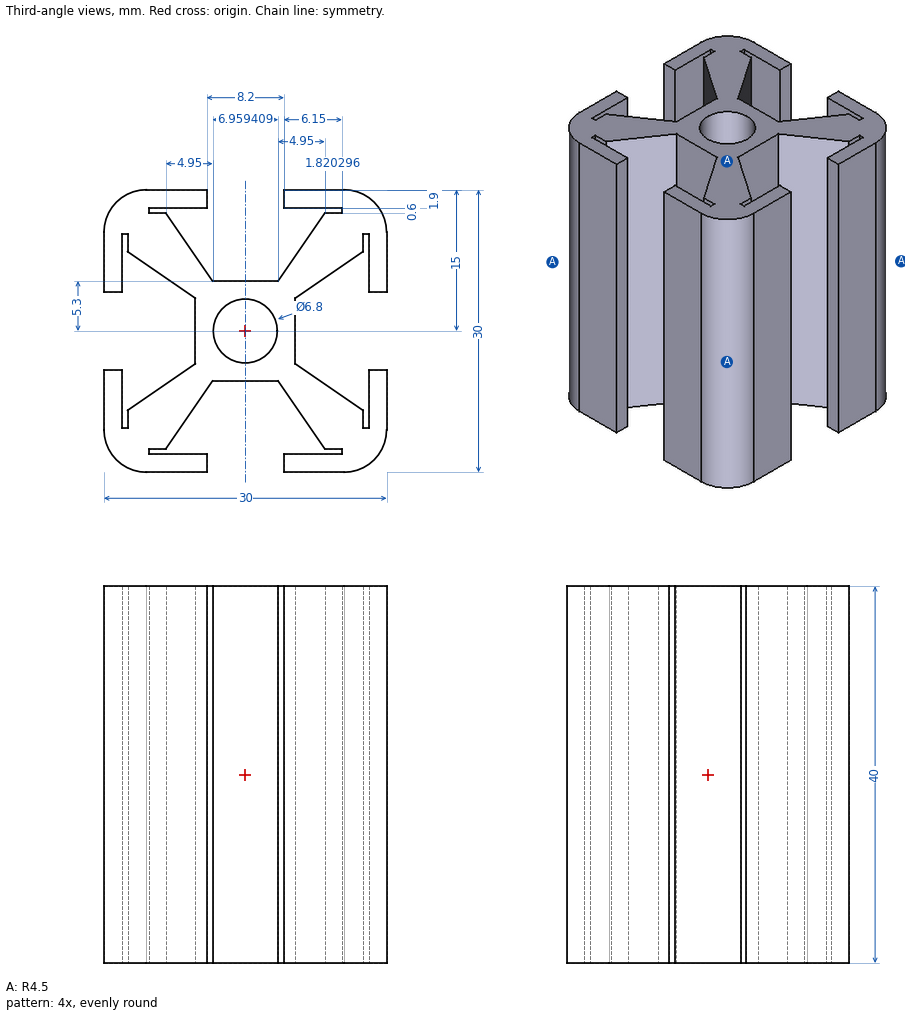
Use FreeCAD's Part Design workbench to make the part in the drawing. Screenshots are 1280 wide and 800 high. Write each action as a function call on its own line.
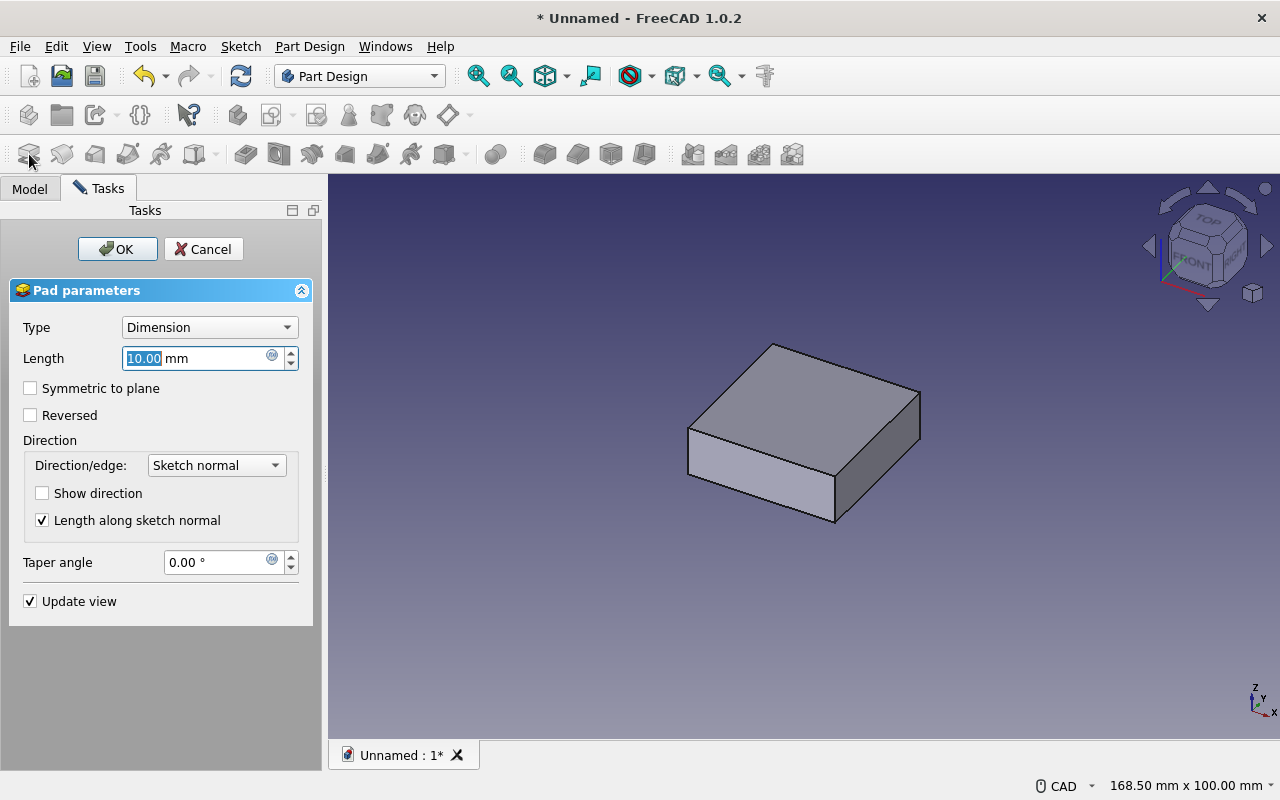
text(40)
key(Tab)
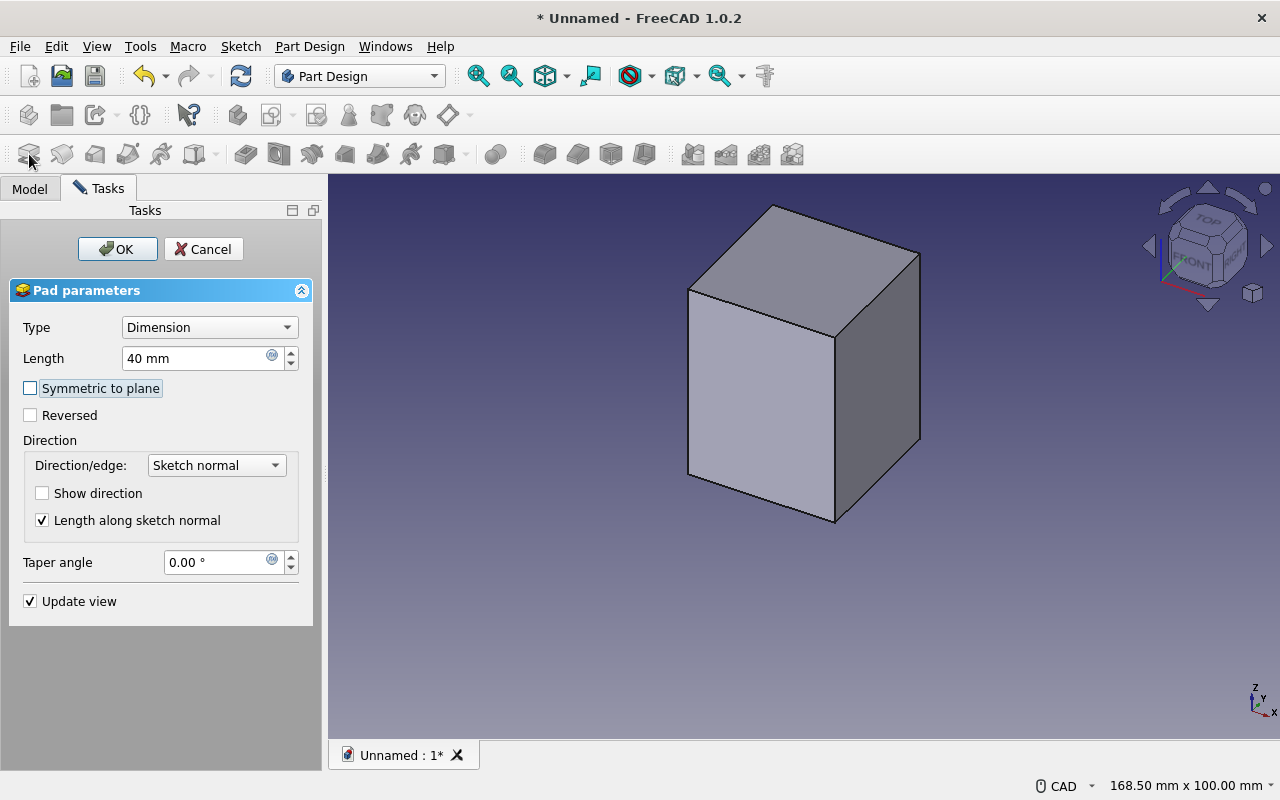
click(31, 388)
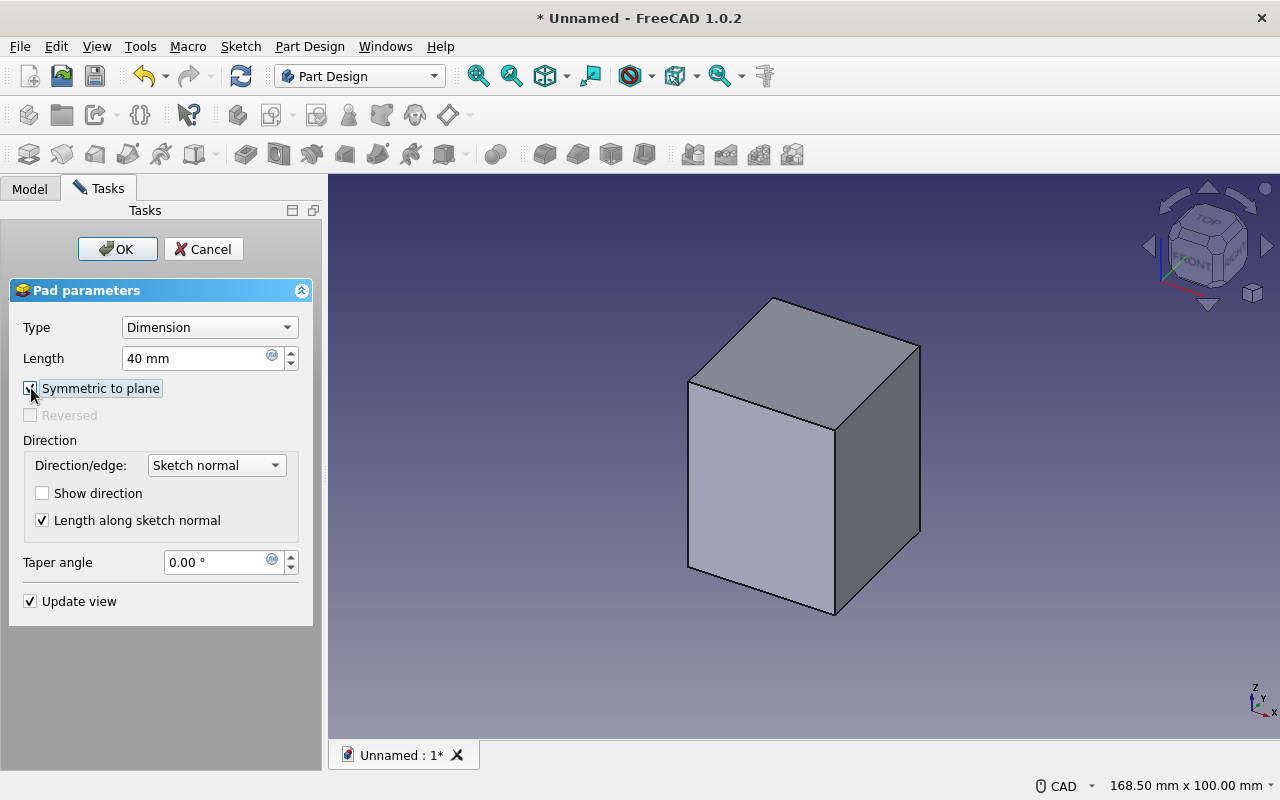
click(118, 249)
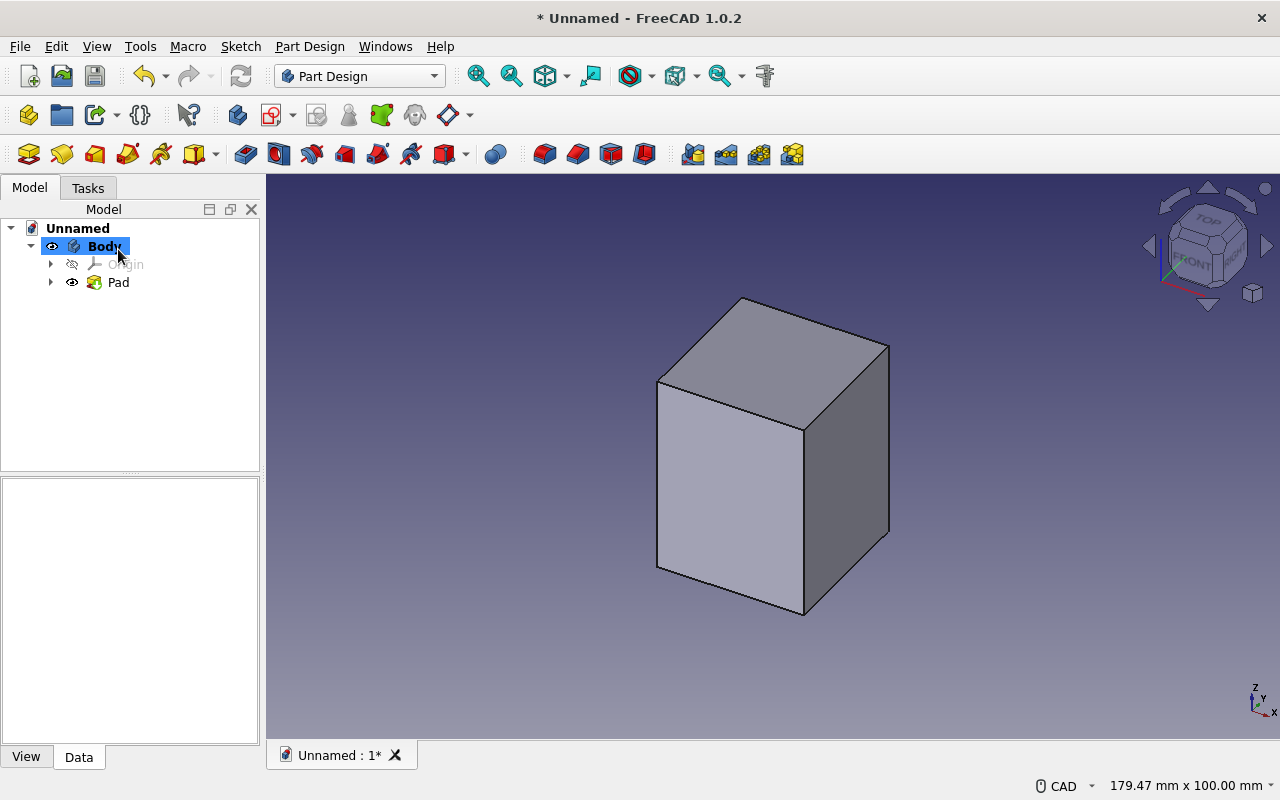
click(804, 522)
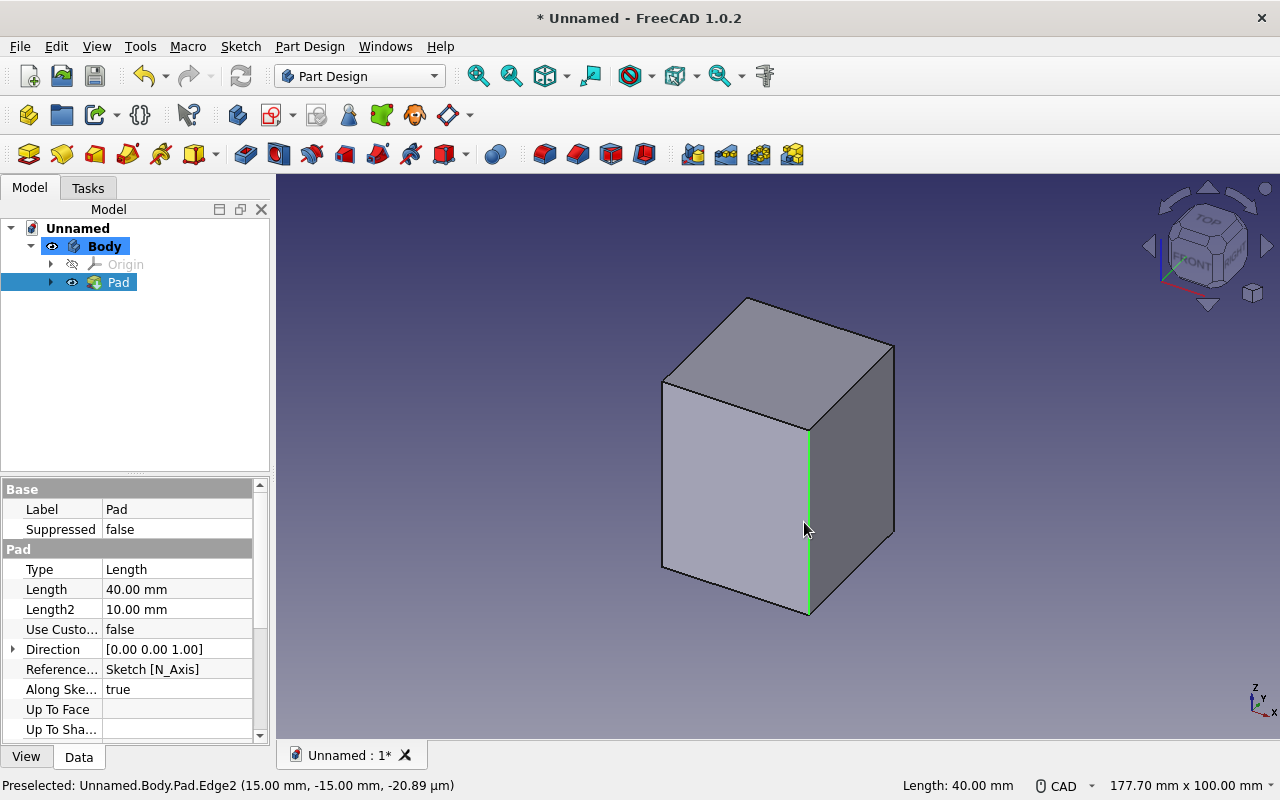
key(0)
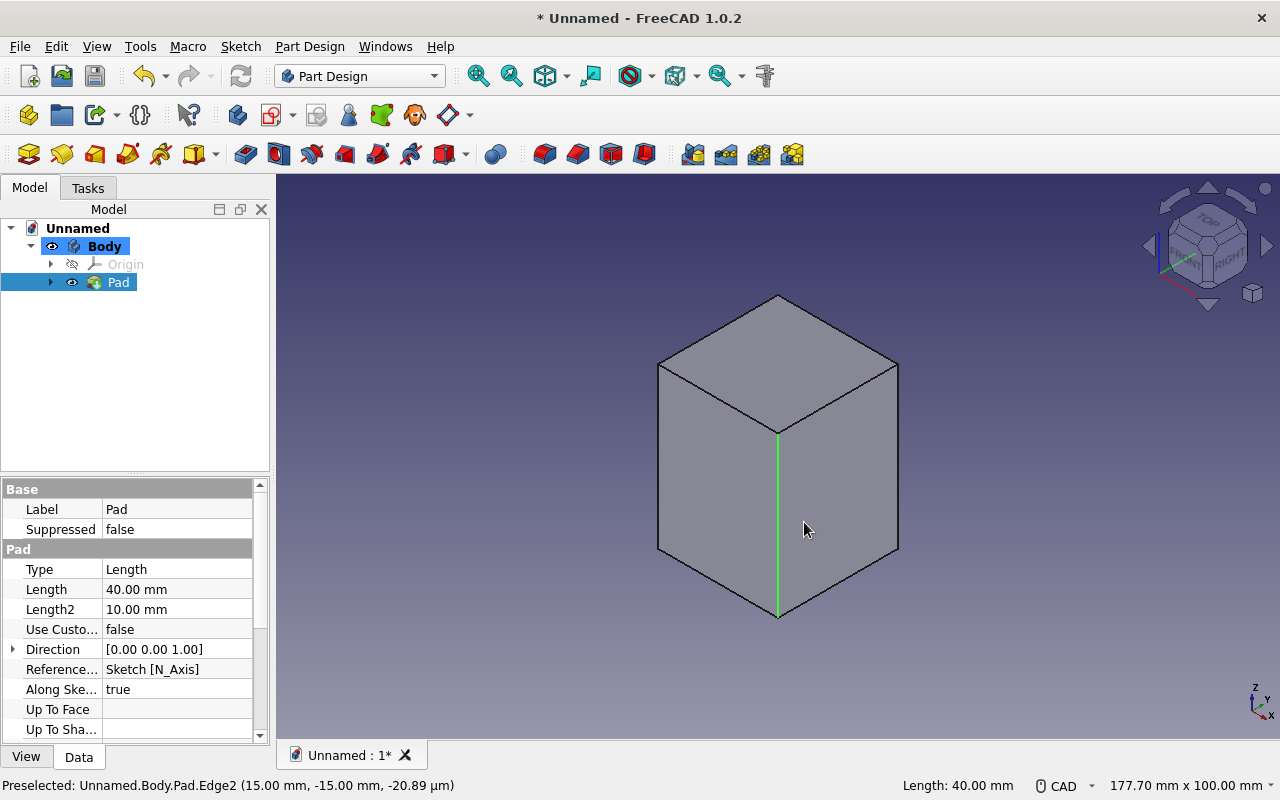
key(2)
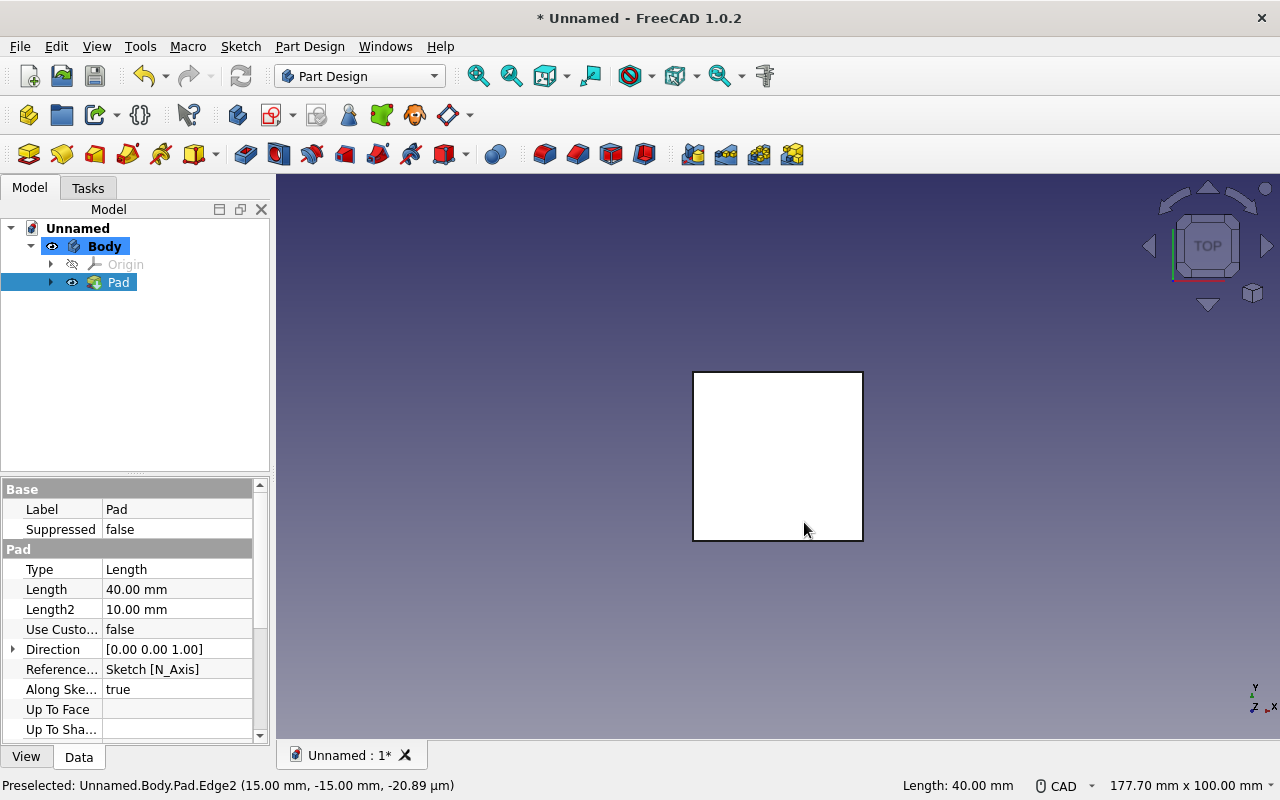
key(v)
key(f)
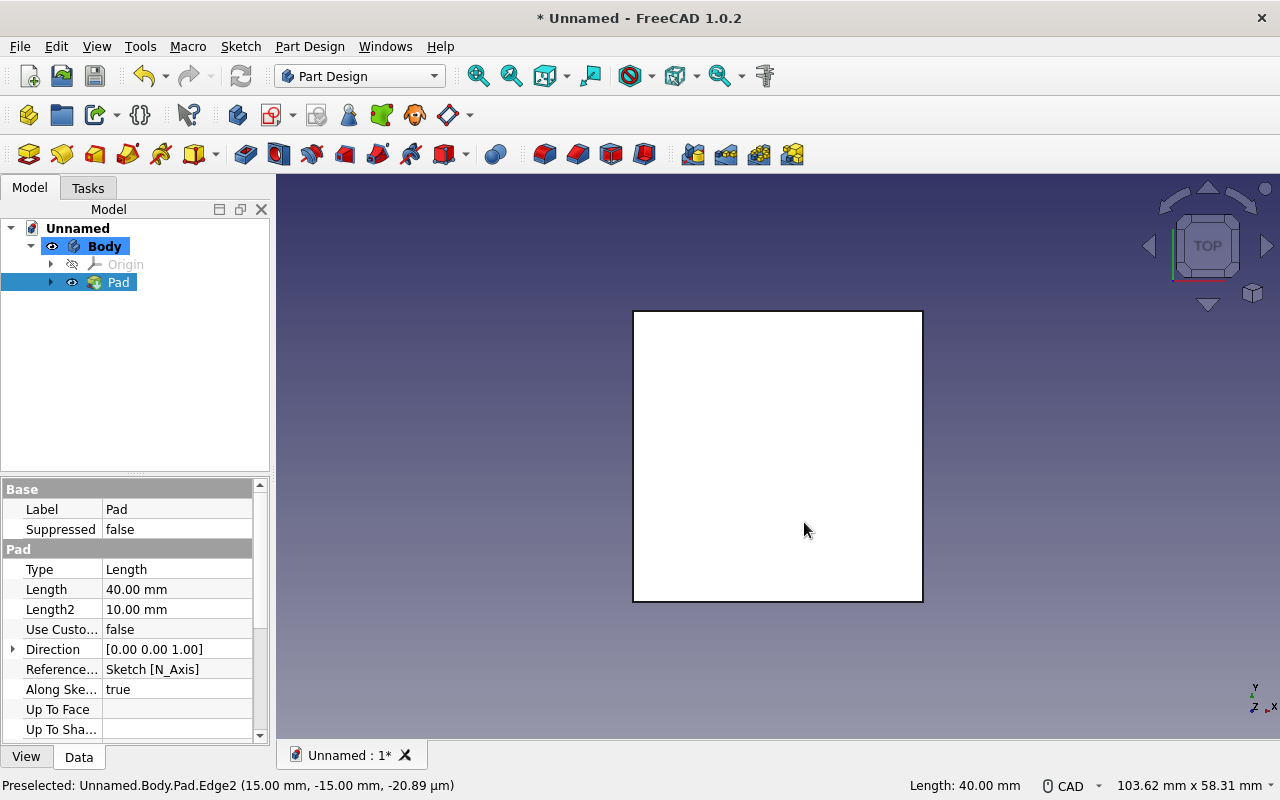
key(1)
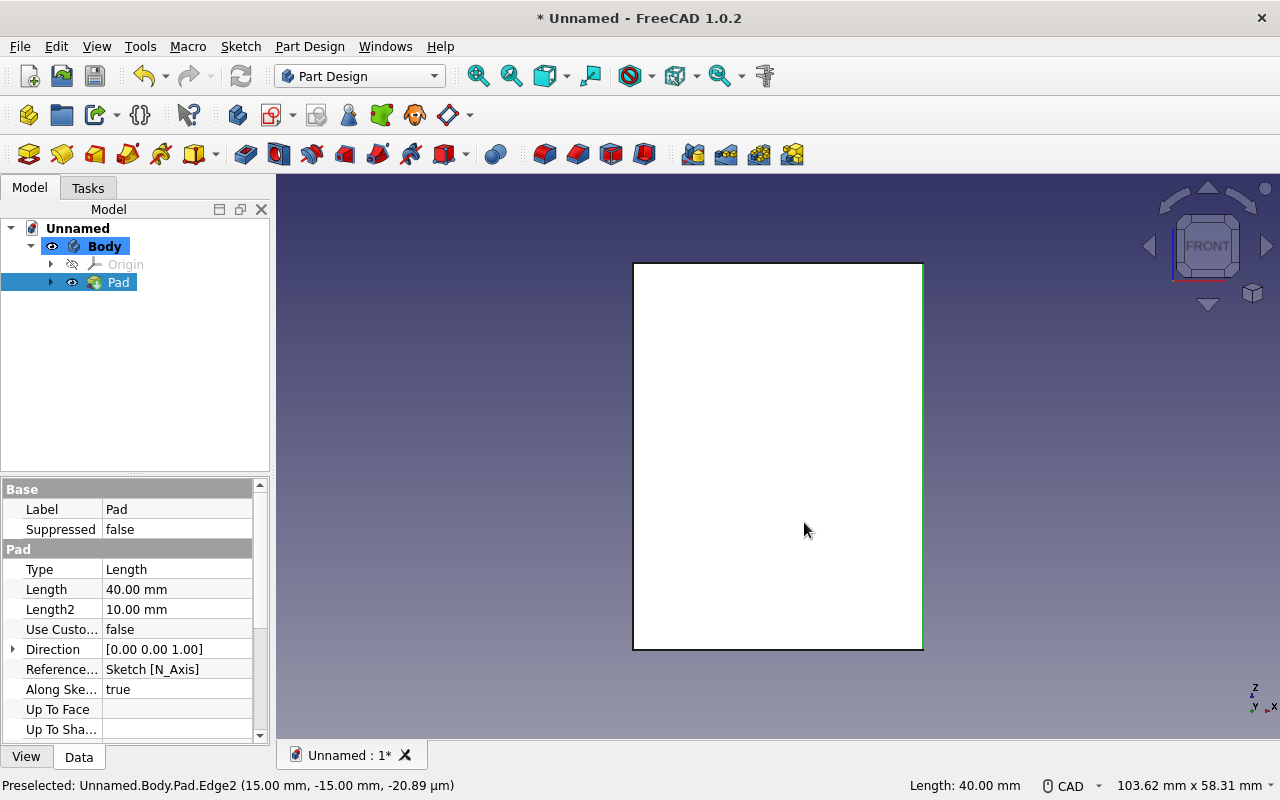
click(633, 456, ctrl)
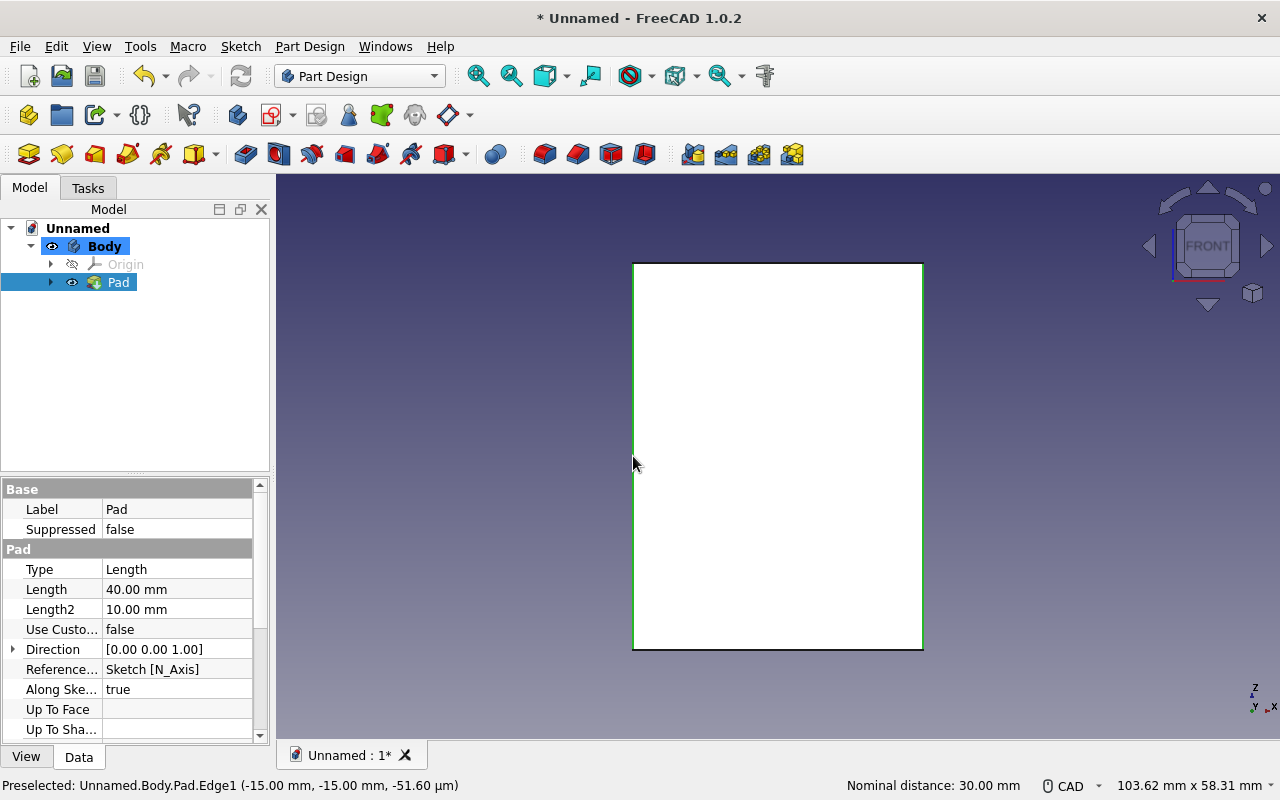
key(3)